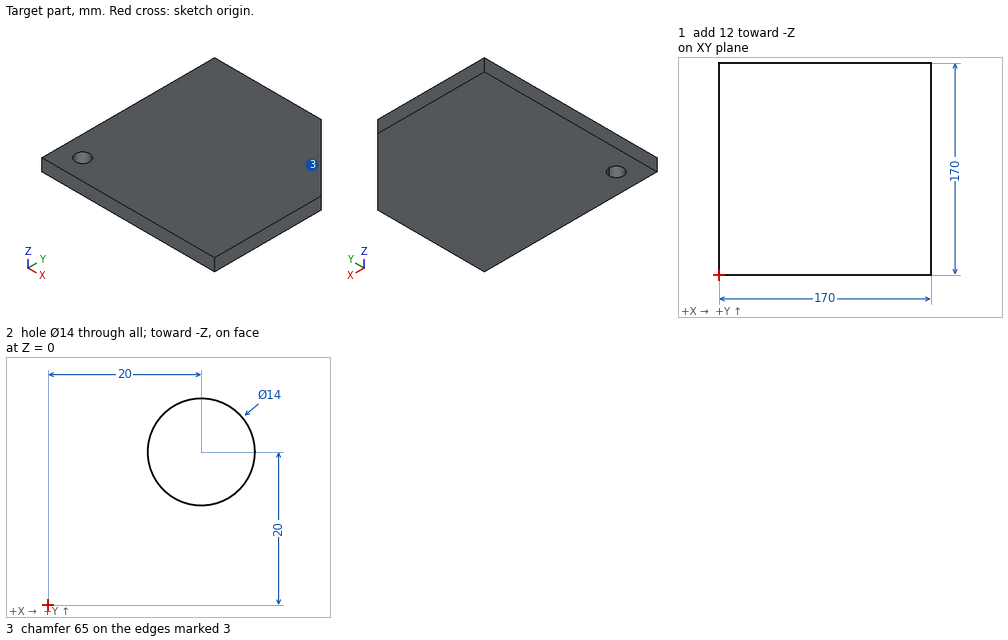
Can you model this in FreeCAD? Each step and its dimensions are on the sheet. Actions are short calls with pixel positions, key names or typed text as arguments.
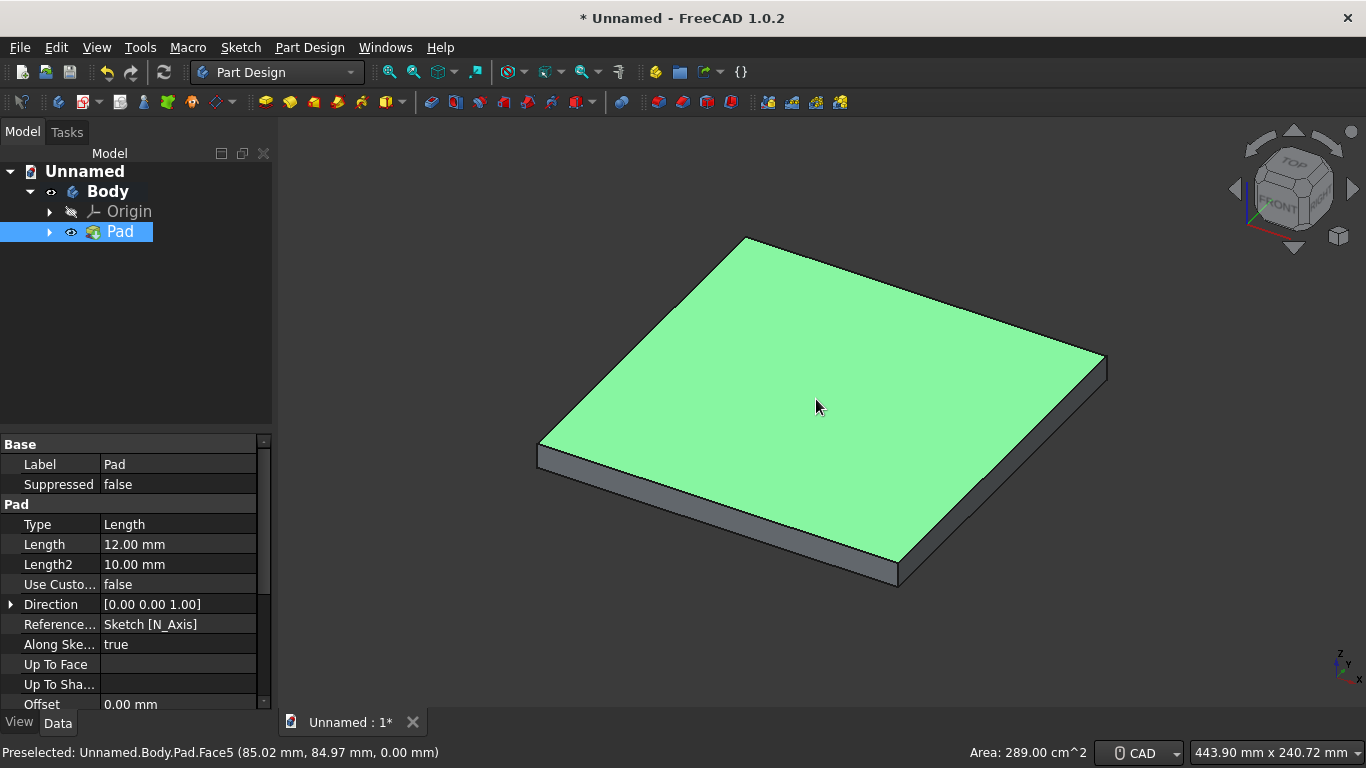
click(84, 102)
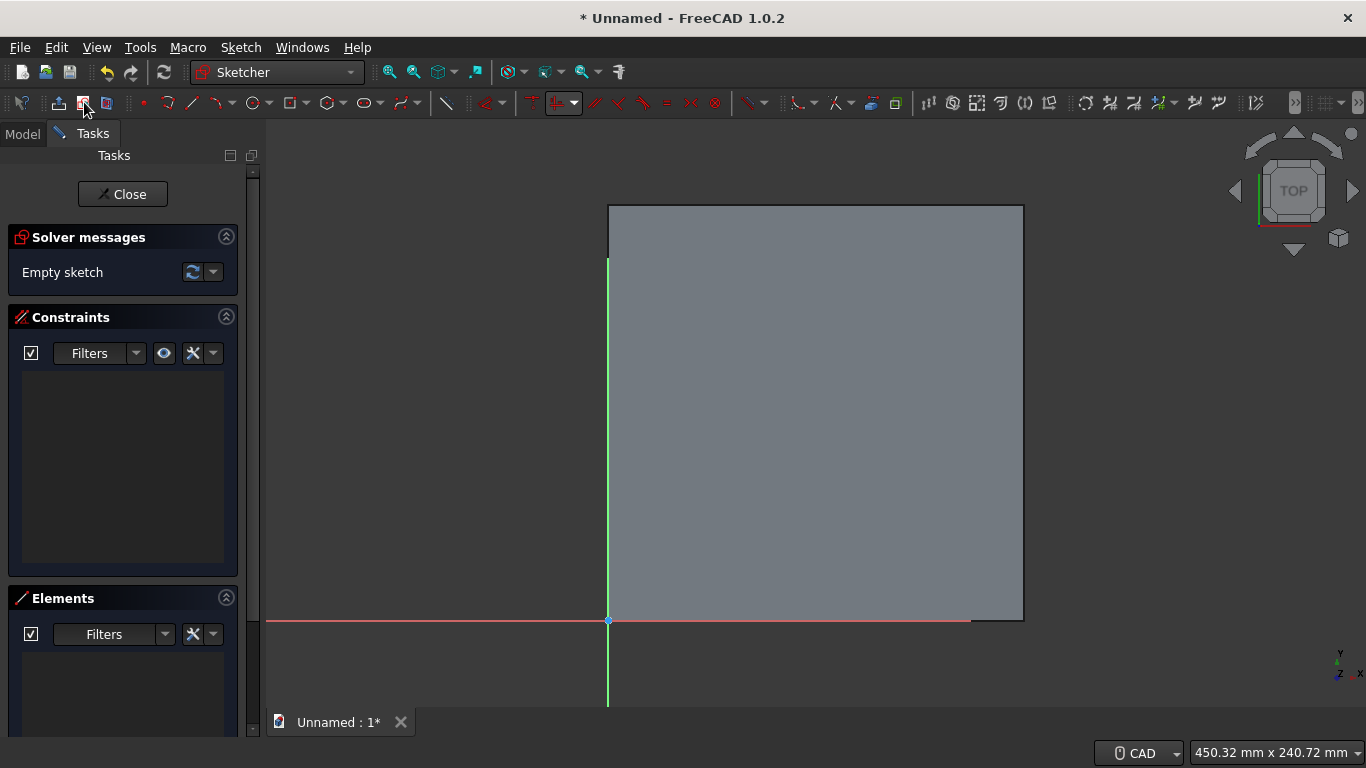
scroll(620, 622, up, 9)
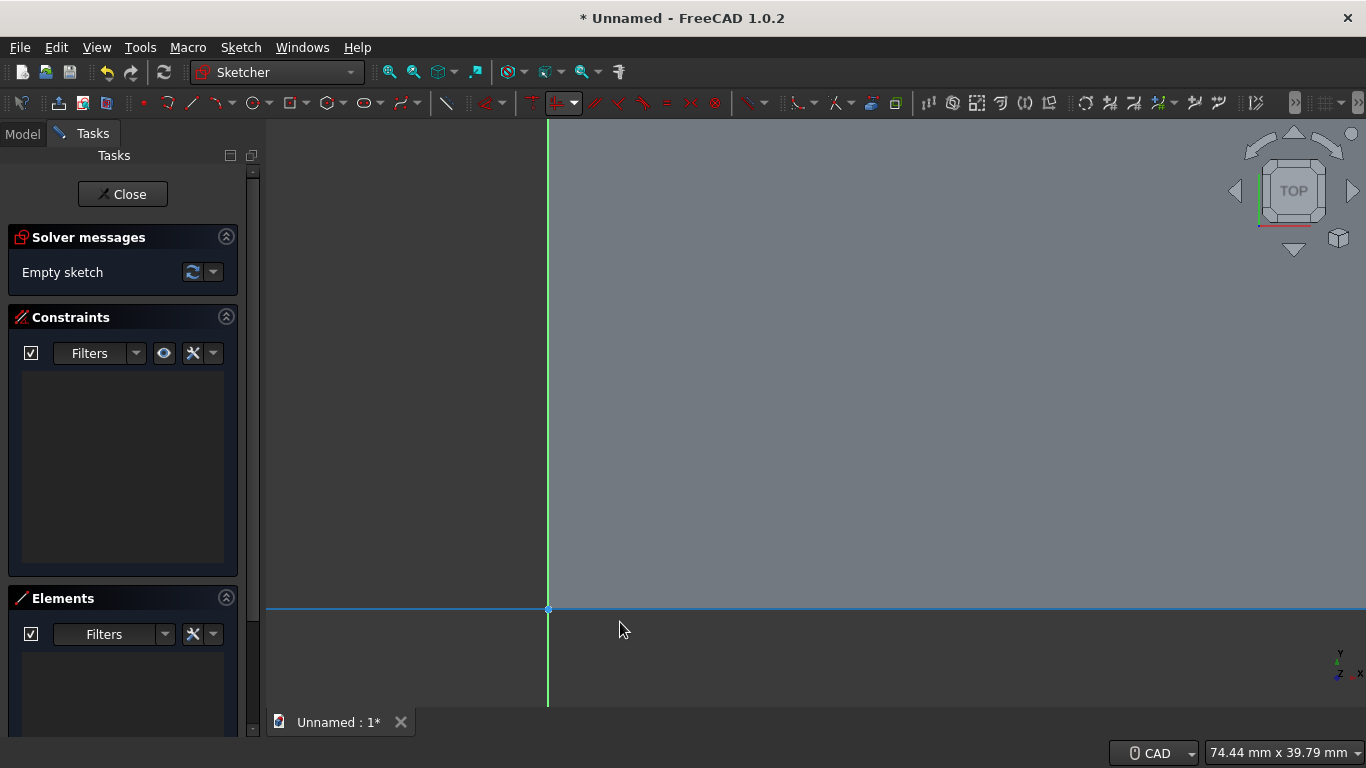
click(254, 104)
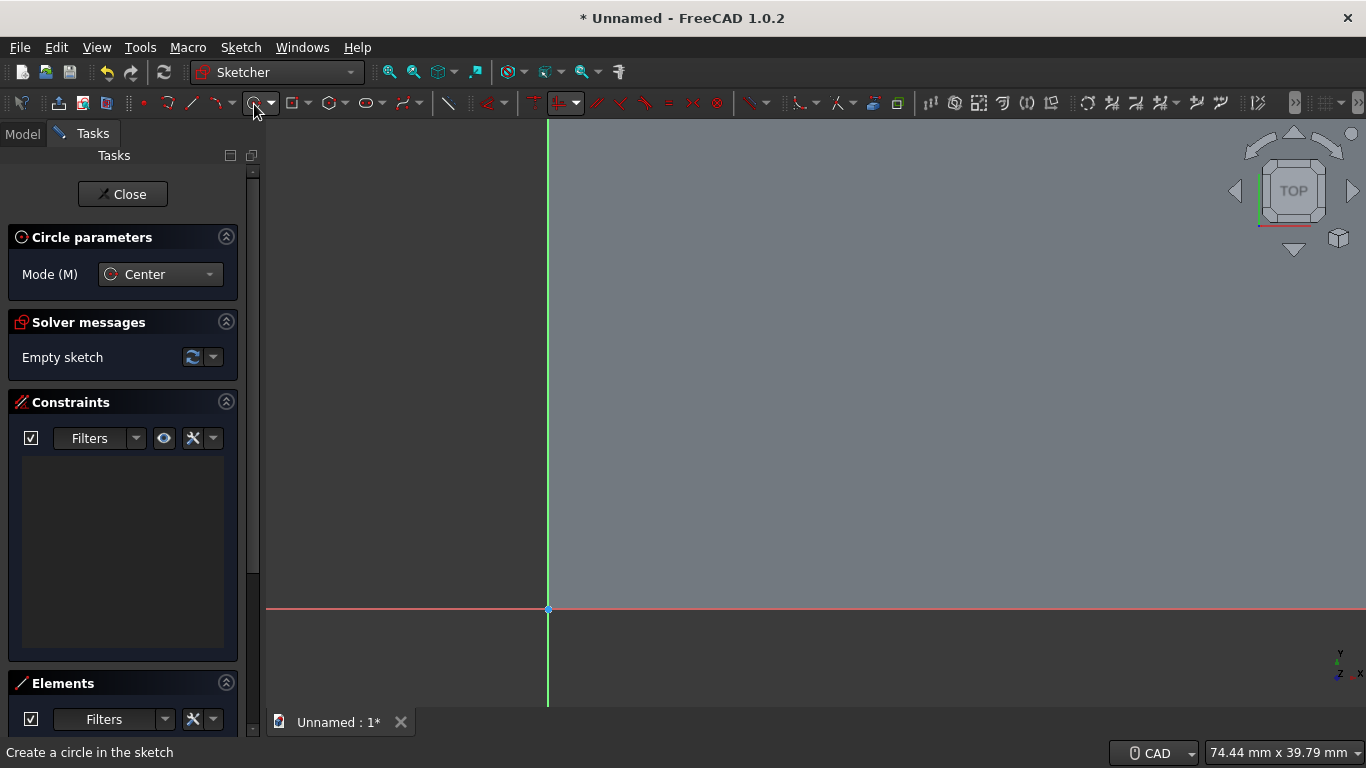
click(844, 314)
click(917, 241)
key(Escape)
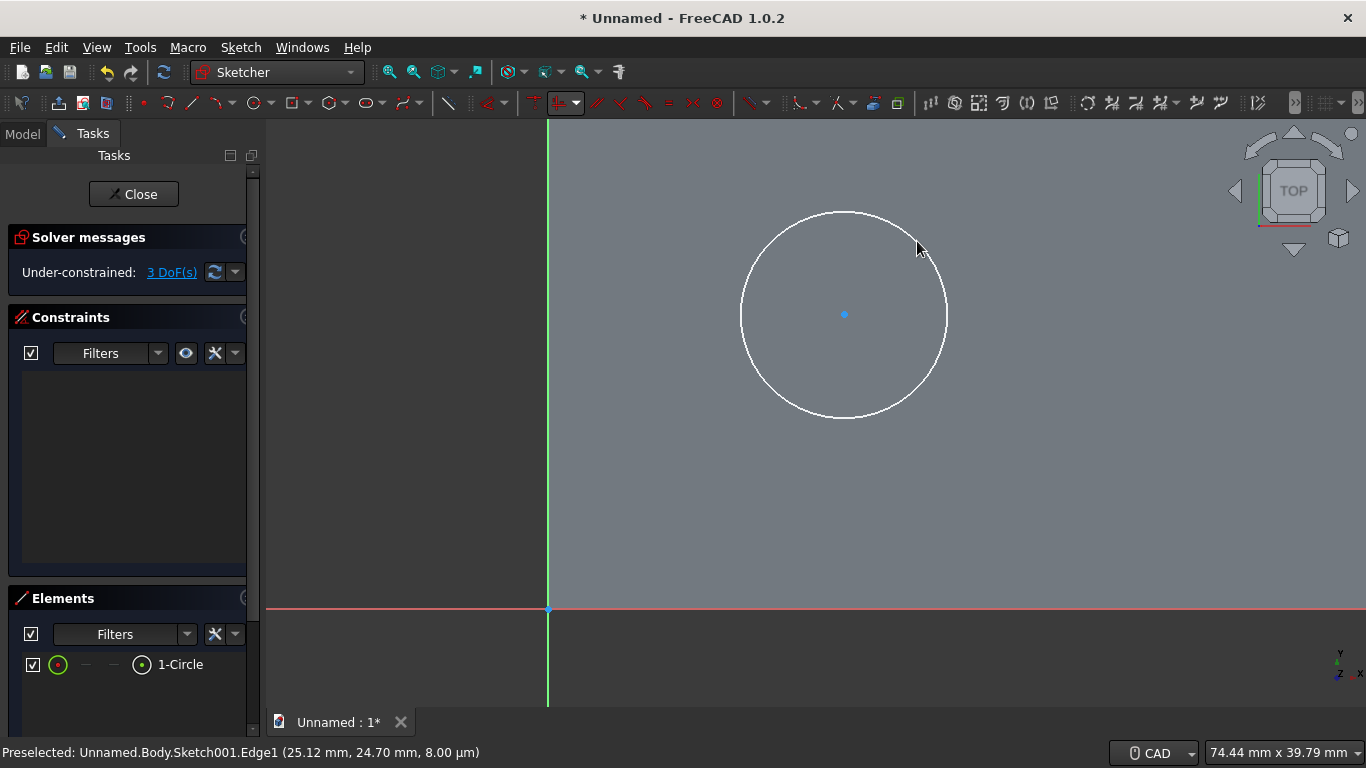
click(917, 242)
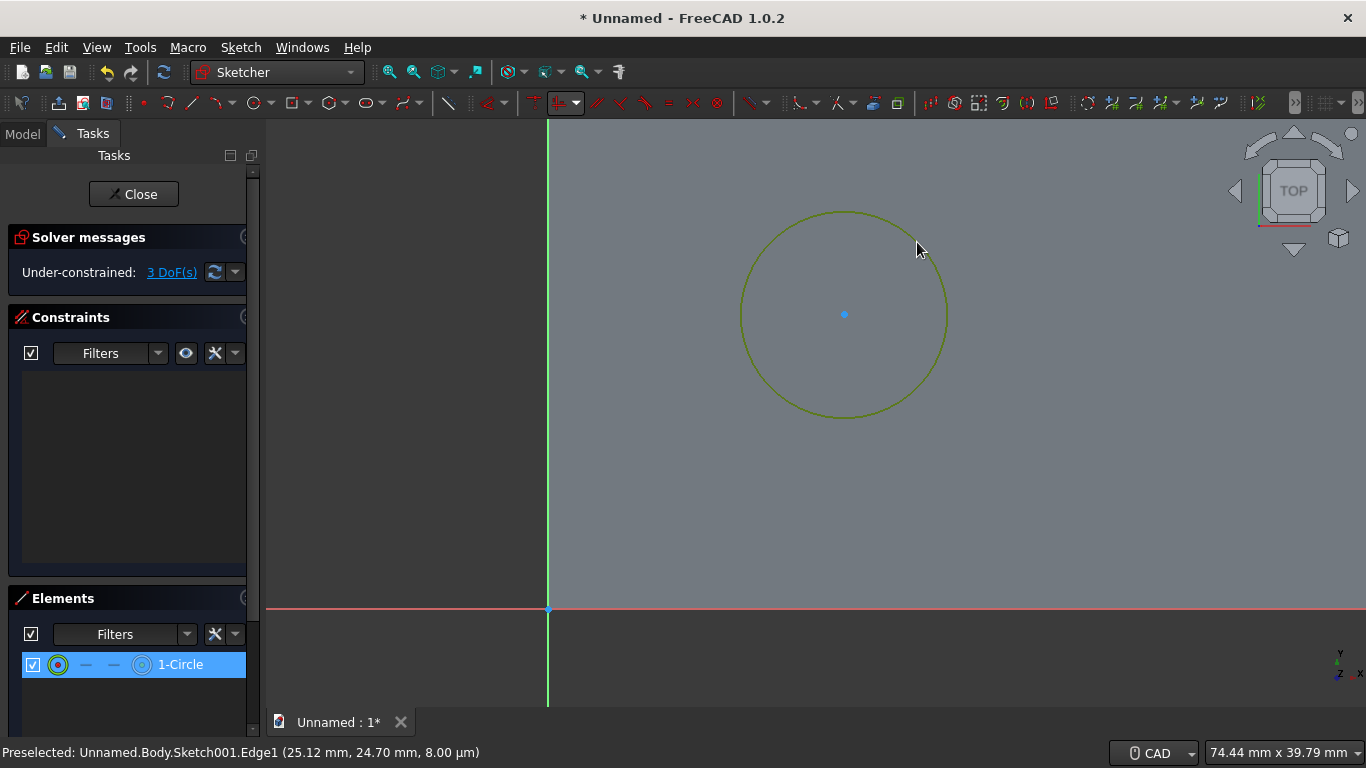
key(k)
key(o)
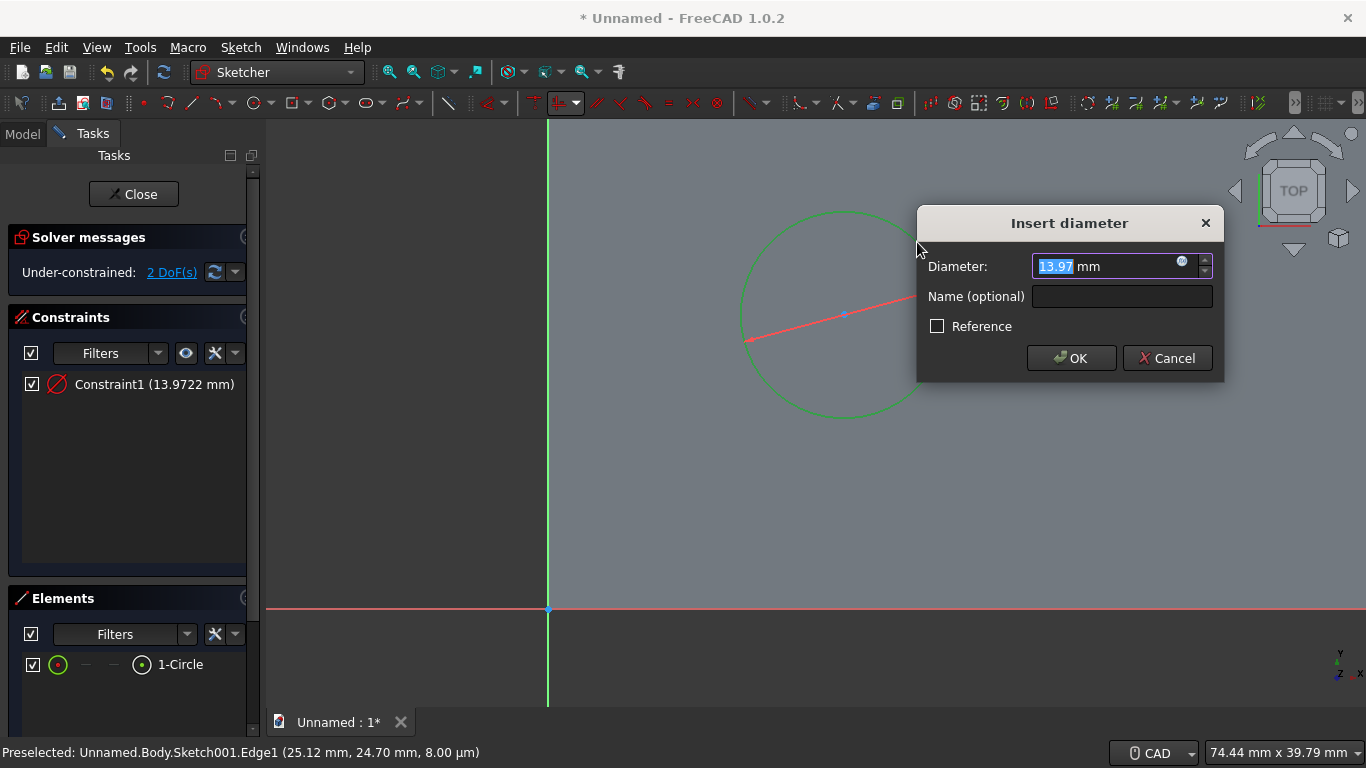
text(14)
key(Return)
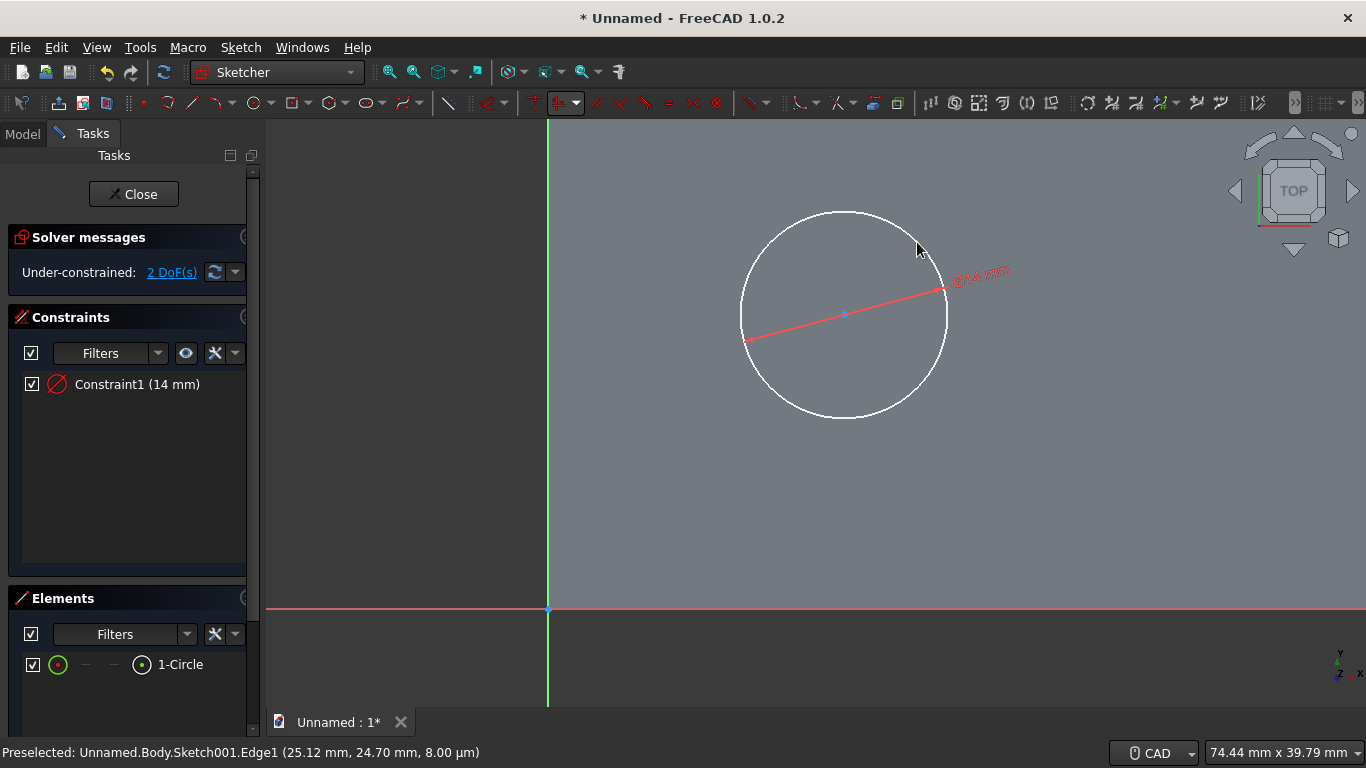
click(844, 315)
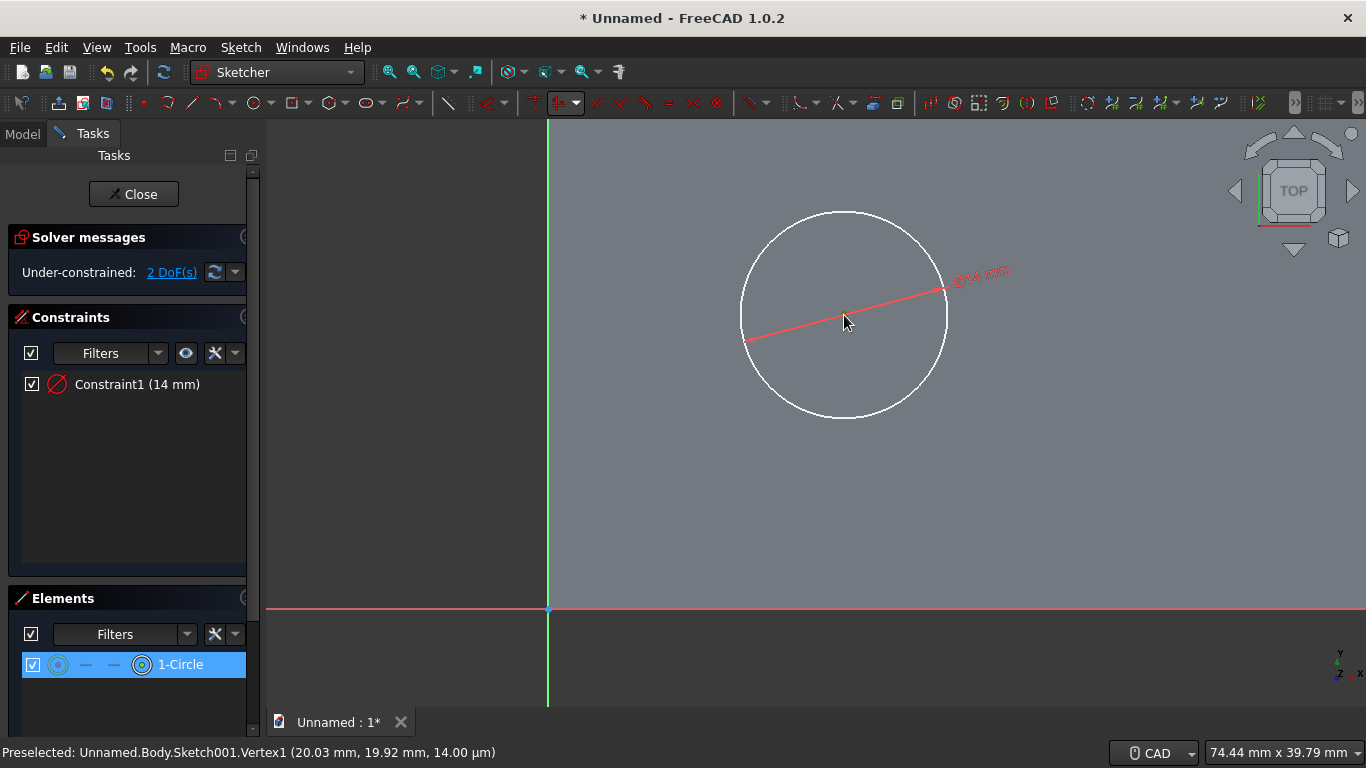
key(l)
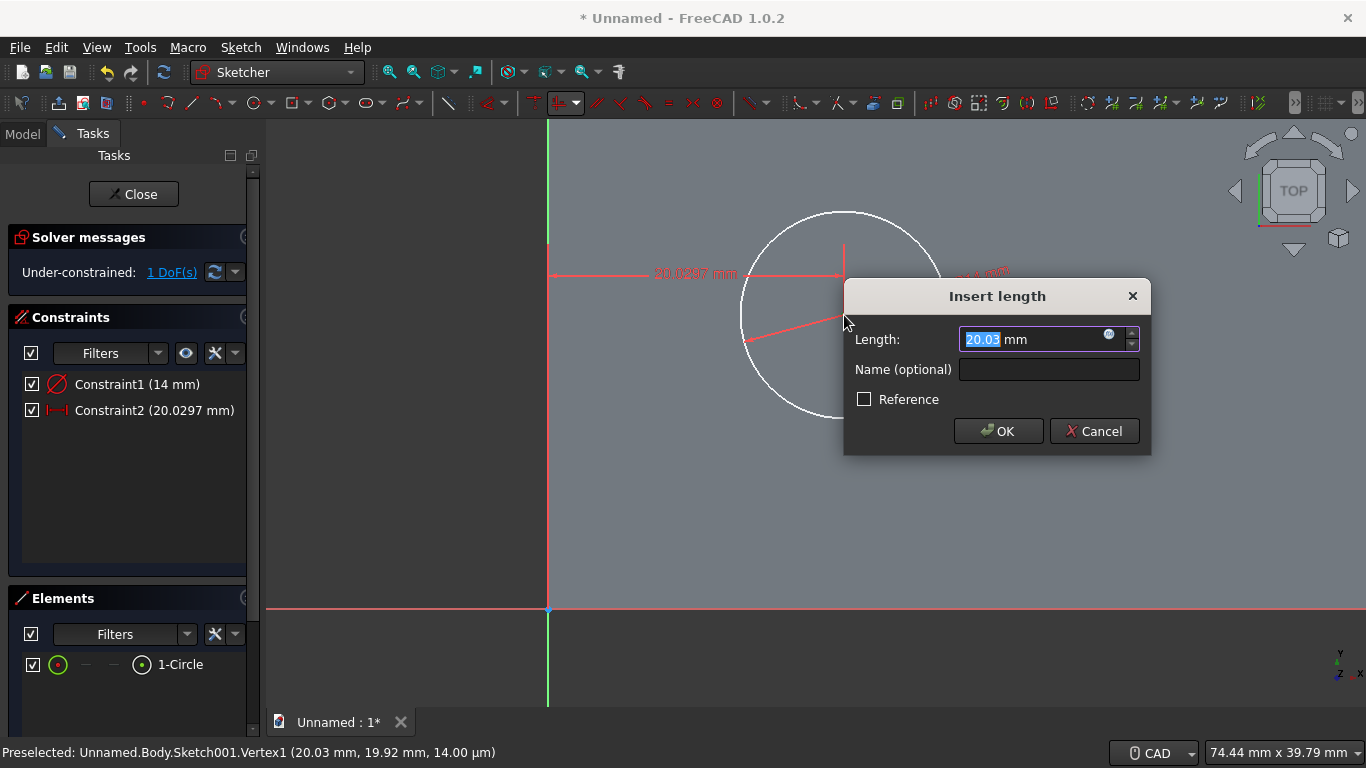
text(20)
key(Return)